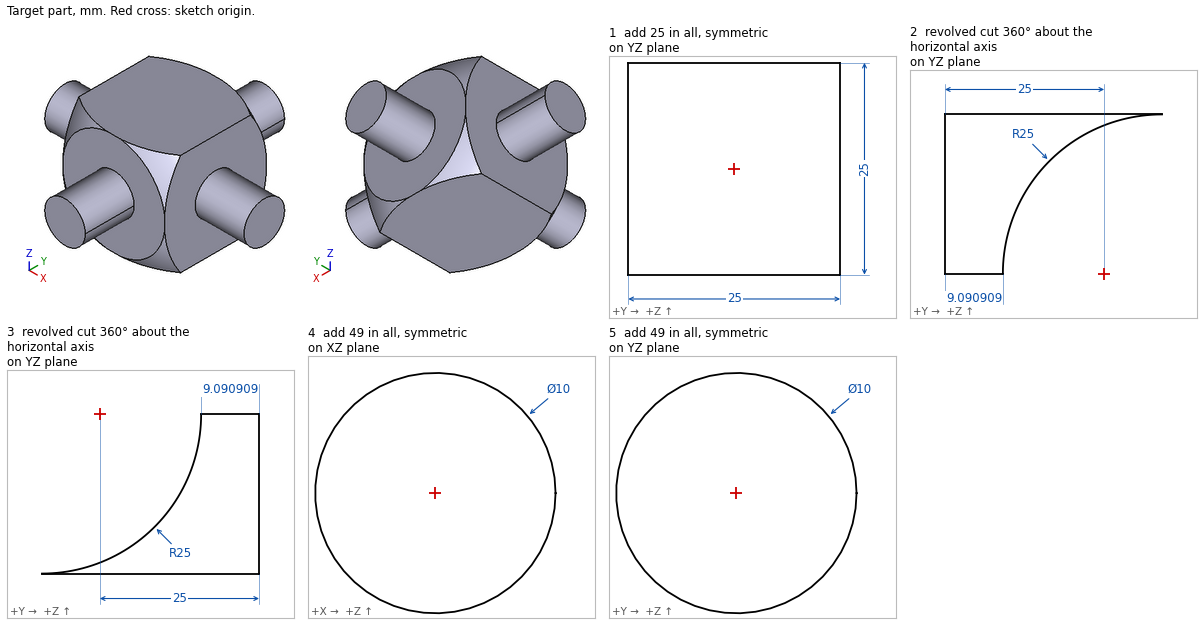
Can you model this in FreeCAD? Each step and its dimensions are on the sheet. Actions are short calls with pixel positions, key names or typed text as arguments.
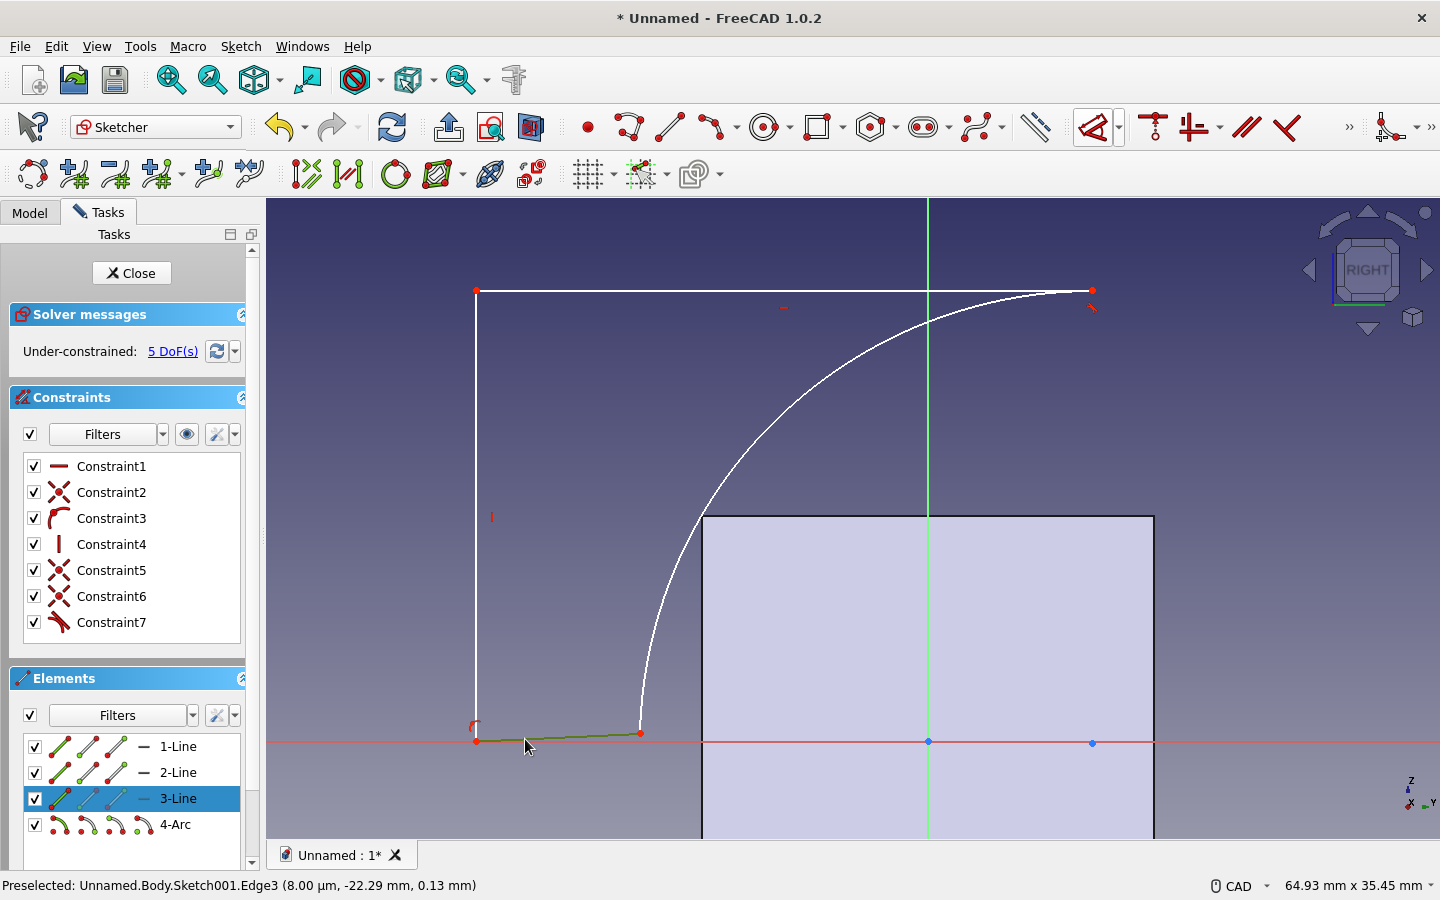
key(h)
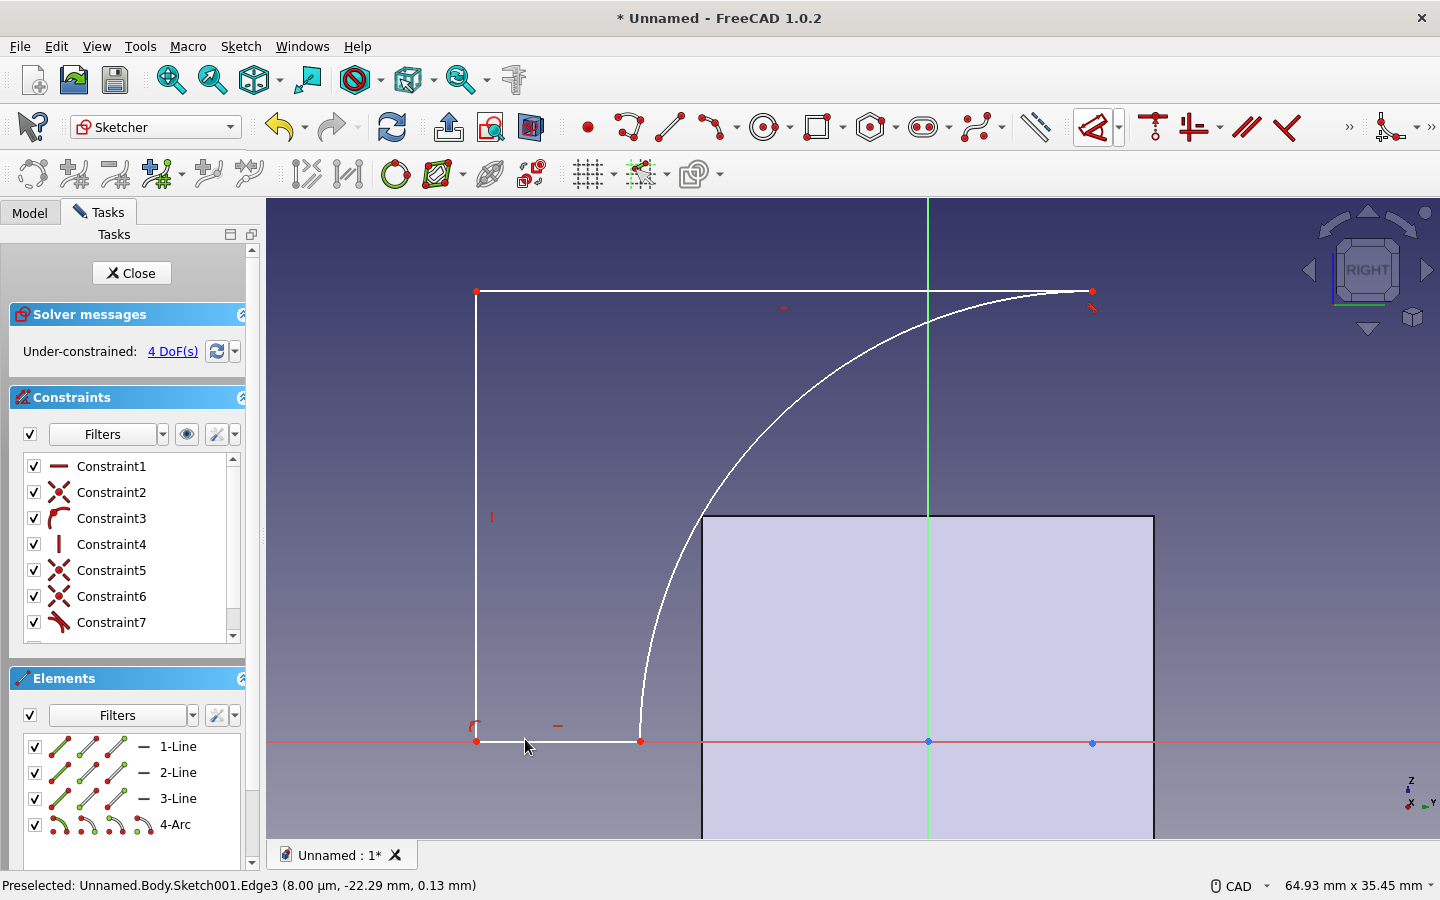
click(1092, 744)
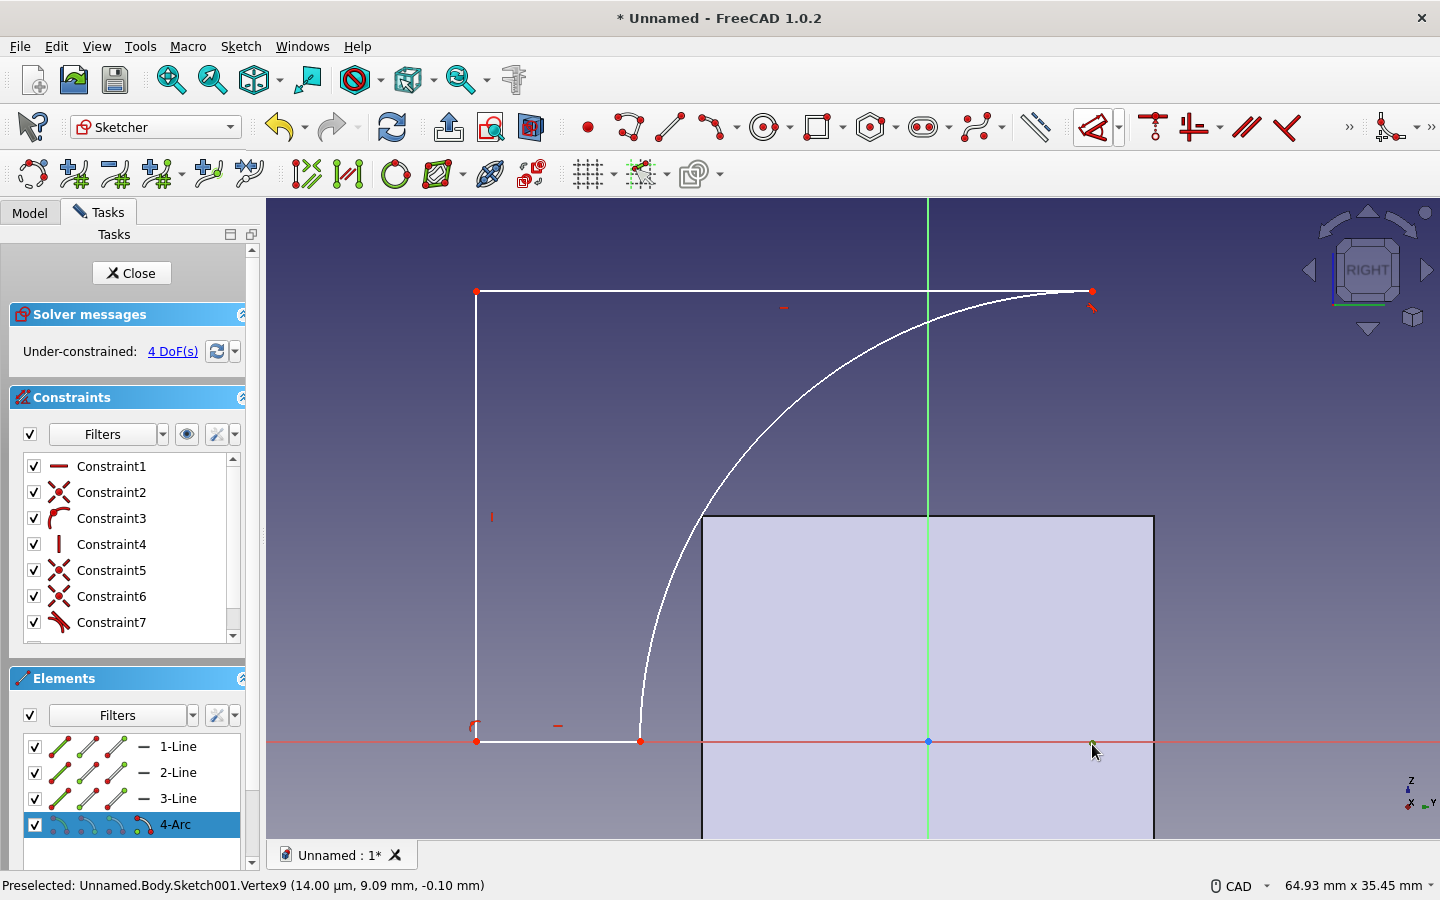
click(364, 742)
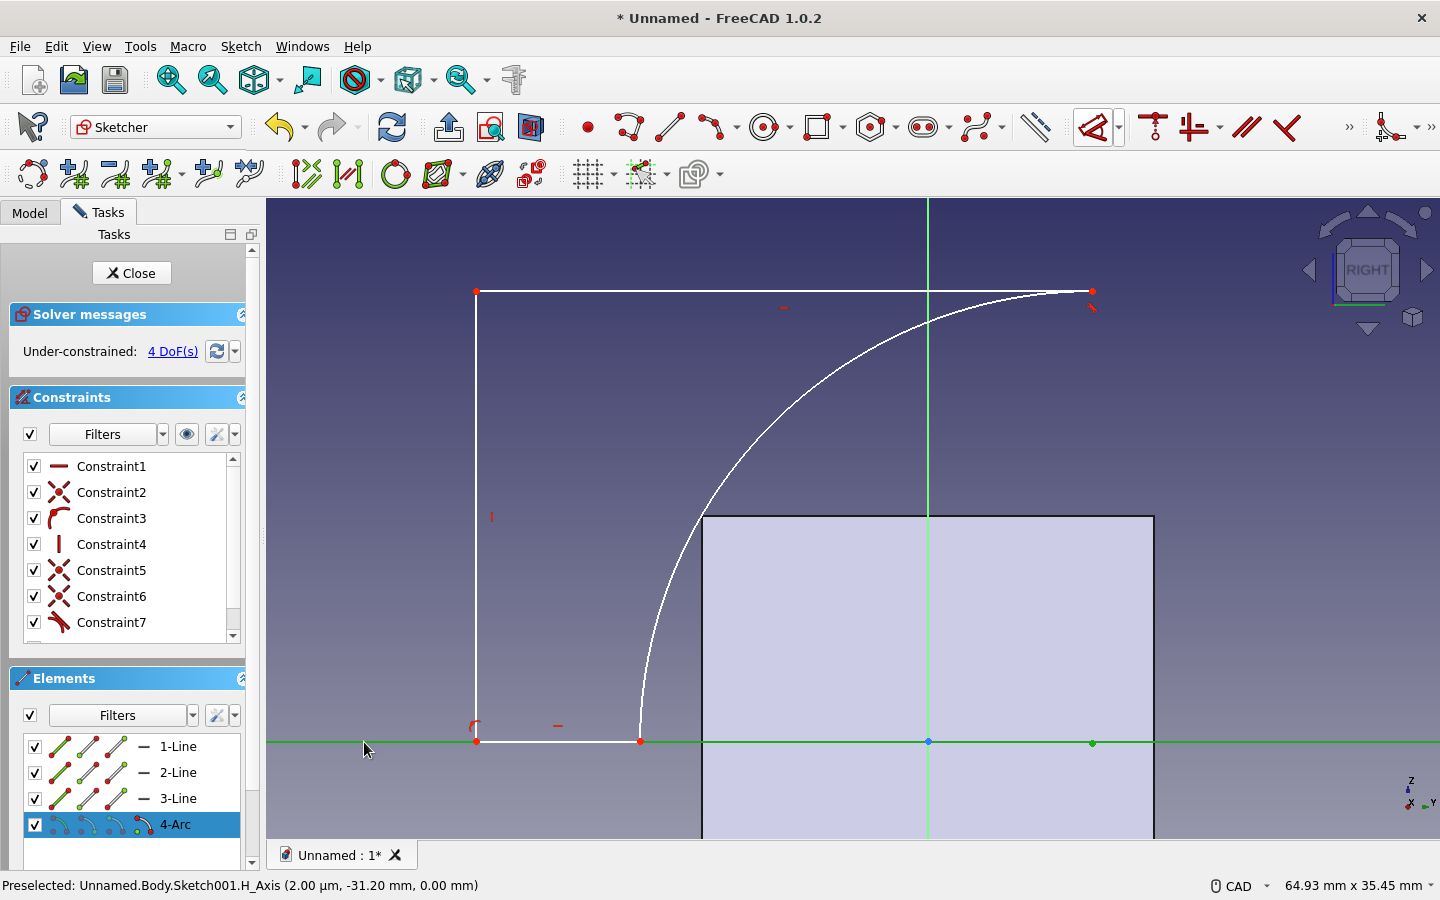
key(c)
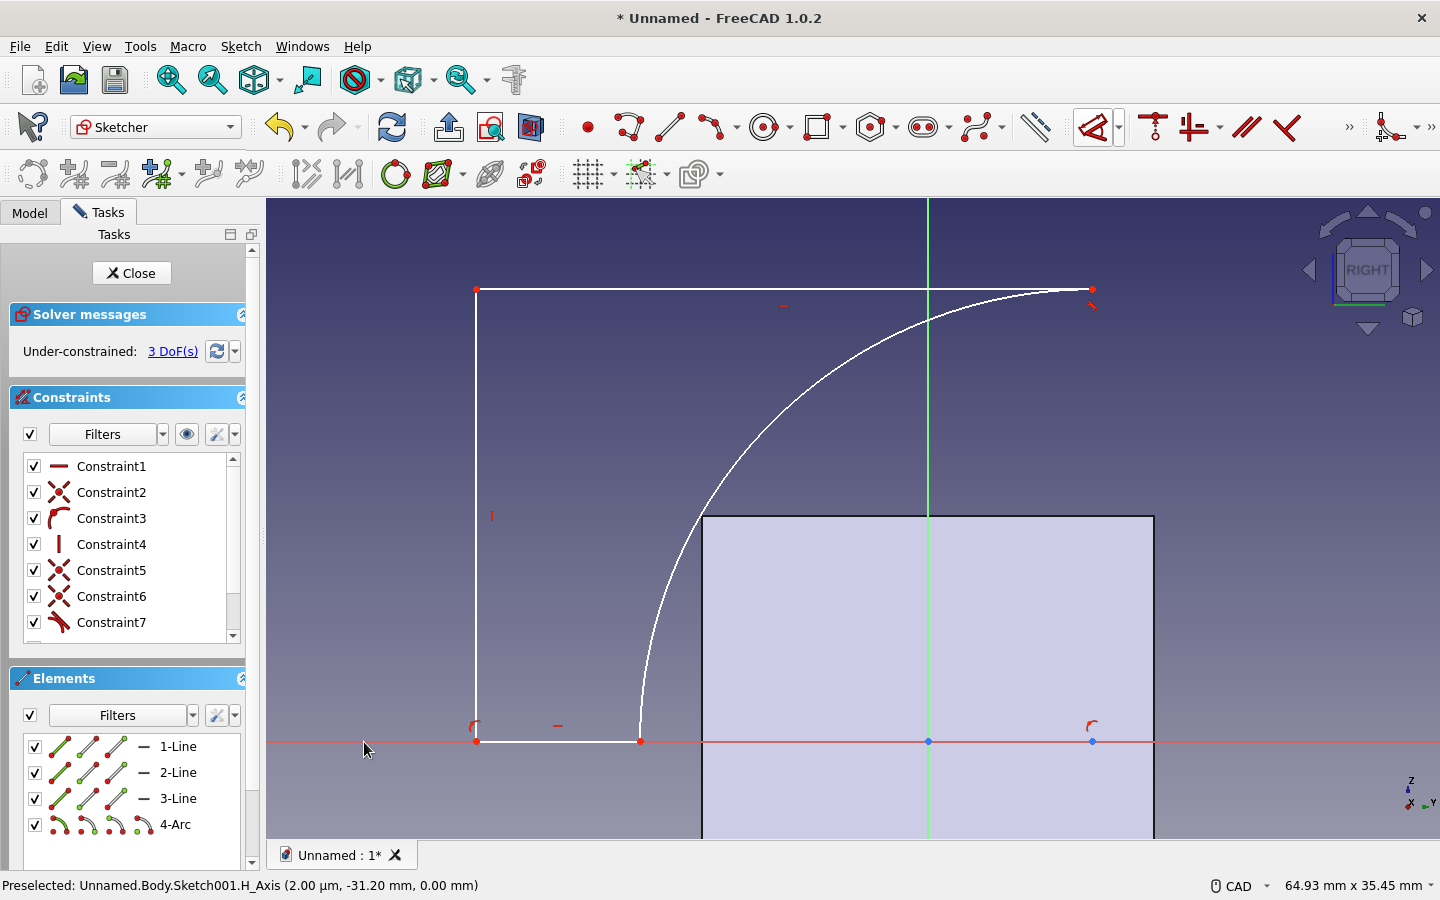
click(1092, 128)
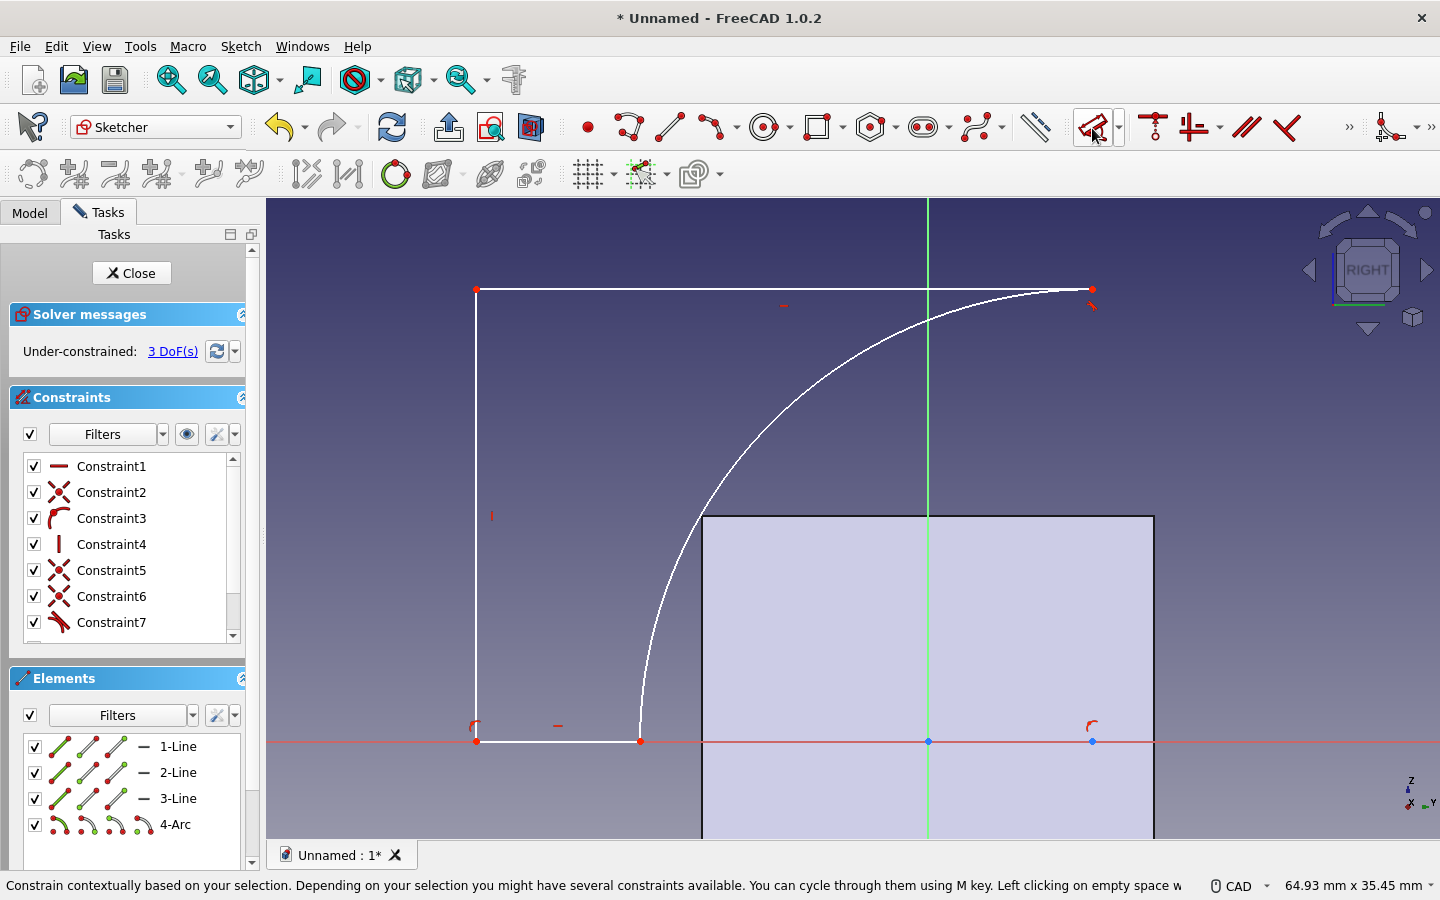
click(887, 339)
click(872, 310)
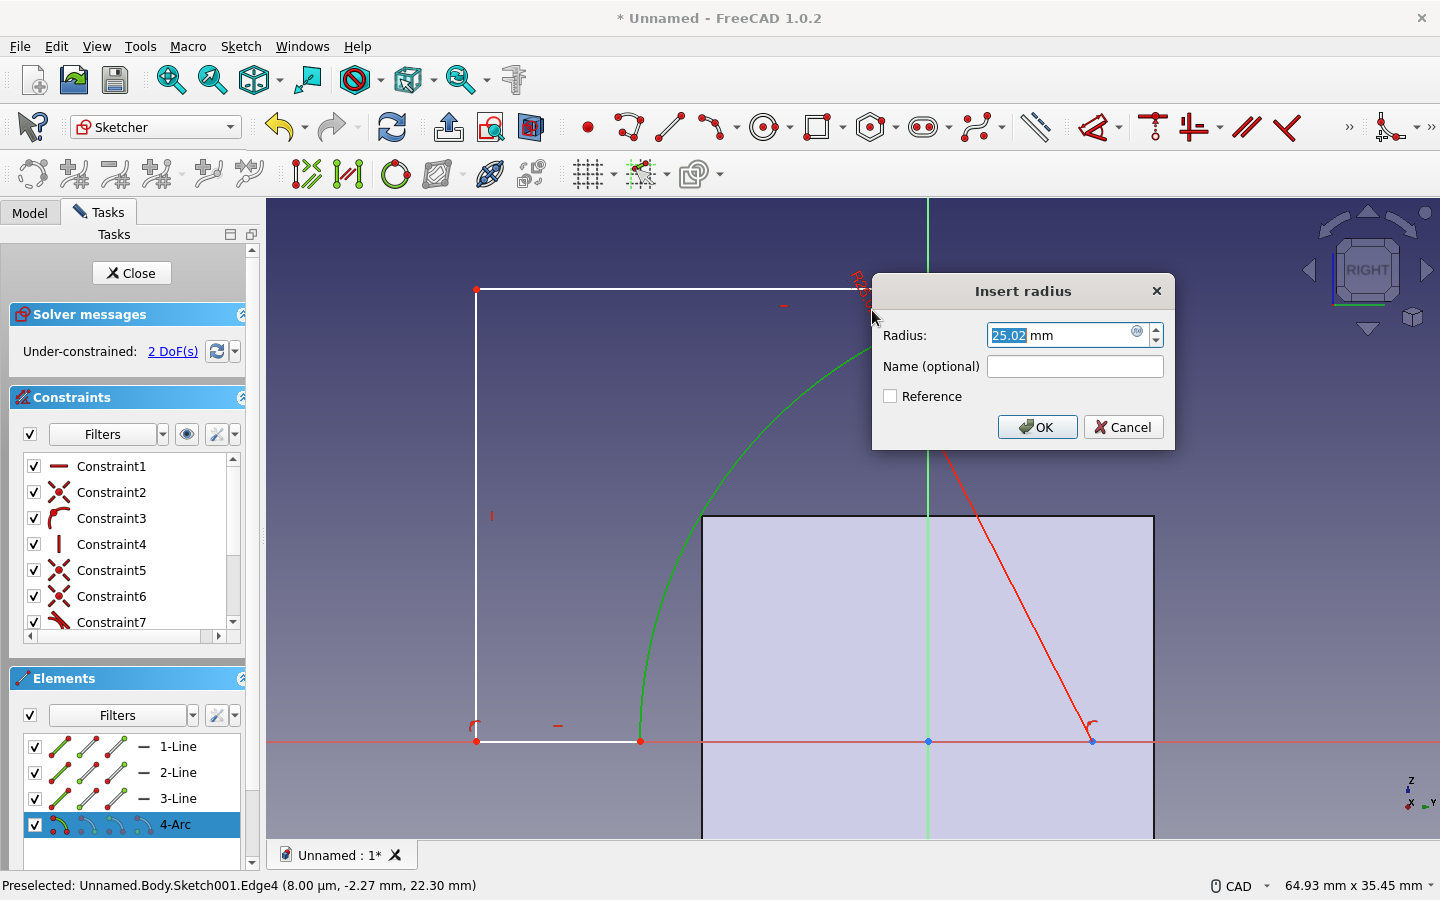
text(25)
key(Return)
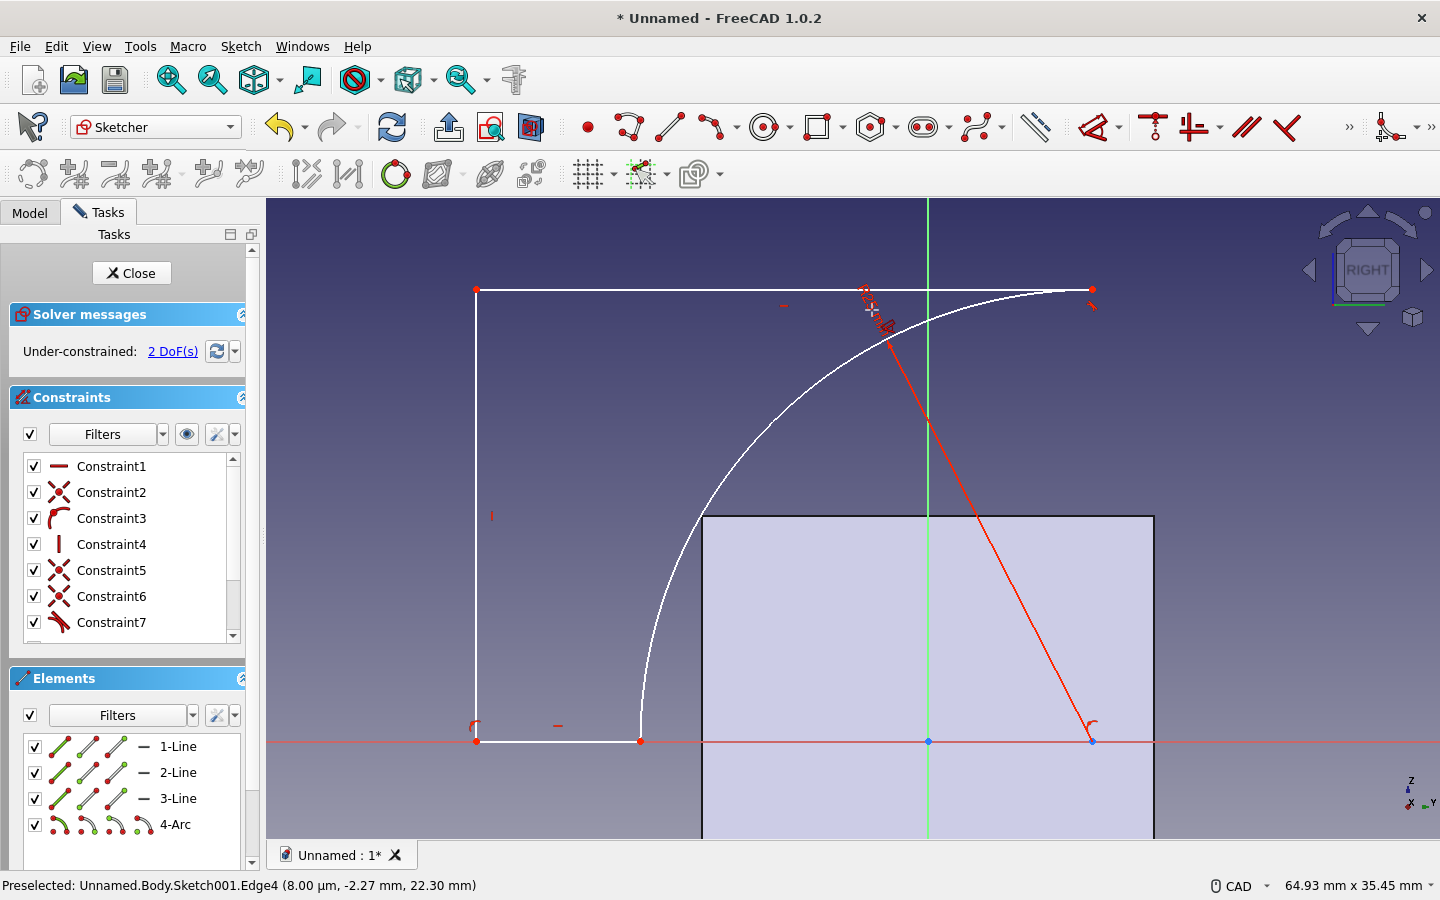
click(476, 290)
click(702, 776)